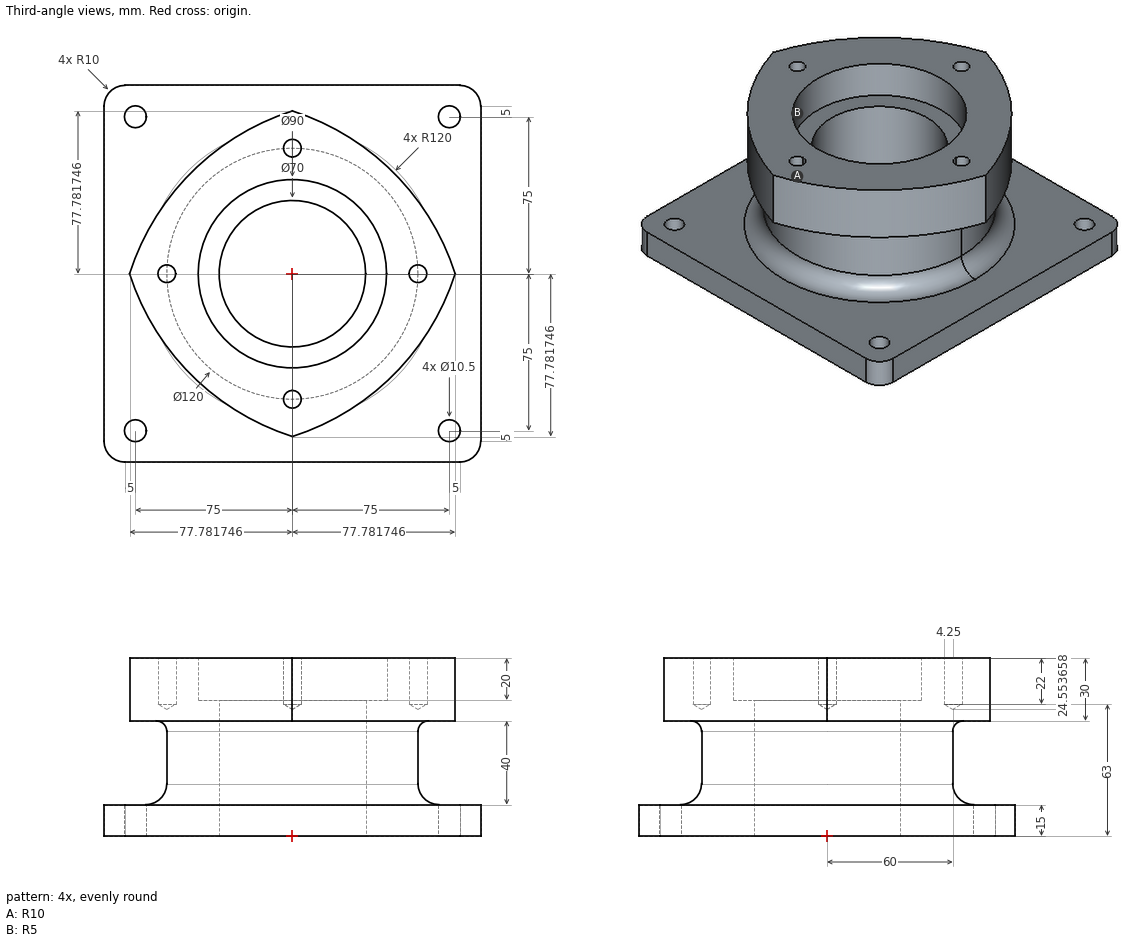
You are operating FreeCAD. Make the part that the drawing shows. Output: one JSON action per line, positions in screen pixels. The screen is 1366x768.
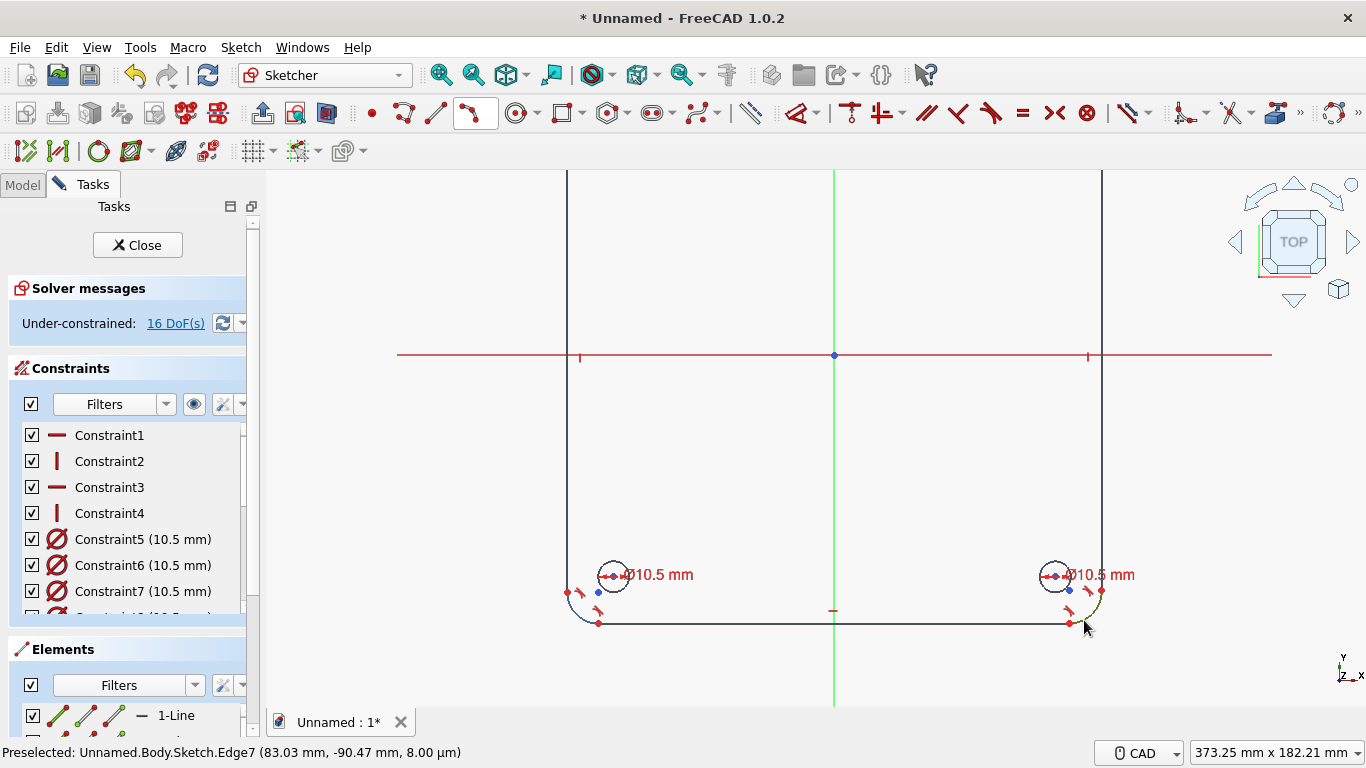
{"action": "scroll", "coordinate": [571, 608], "scroll_direction": "down", "scroll_amount": 2}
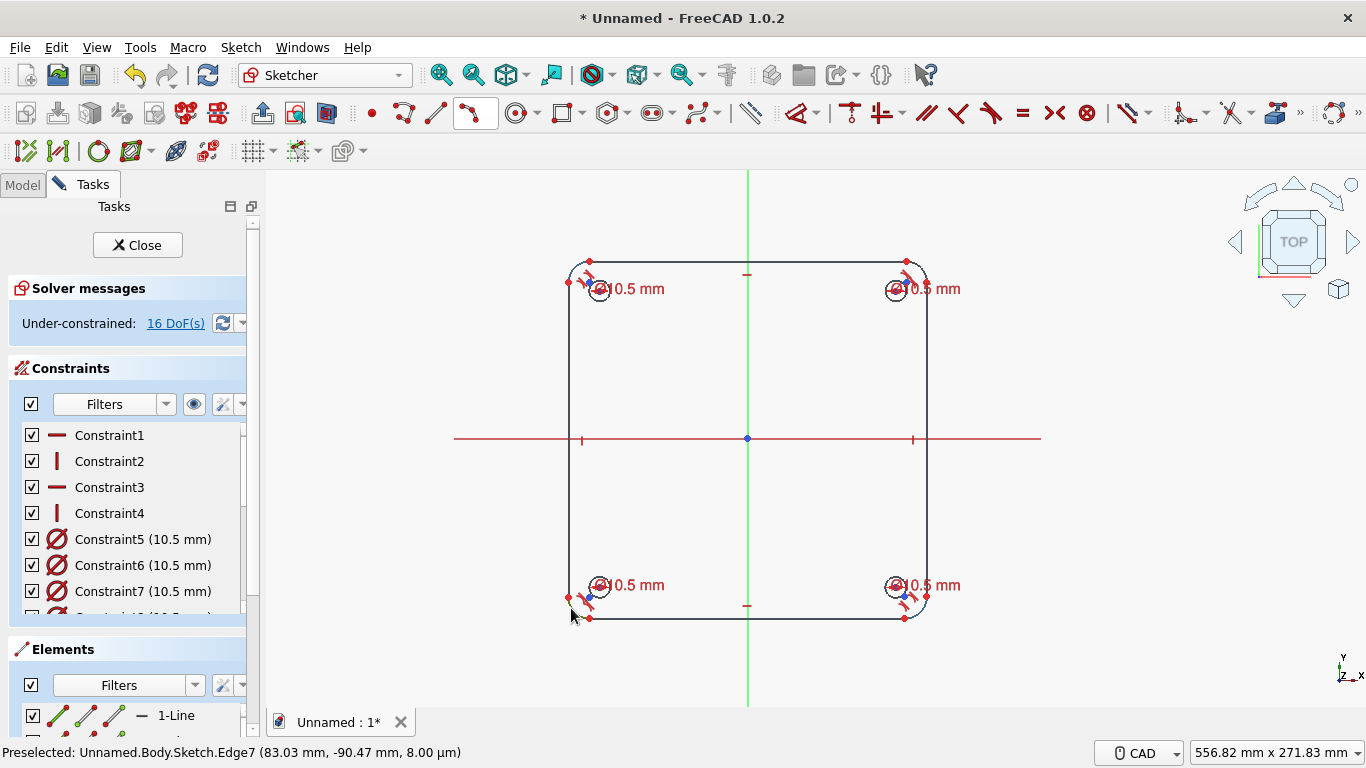
{"action": "scroll", "coordinate": [925, 273], "scroll_direction": "up", "scroll_amount": 2}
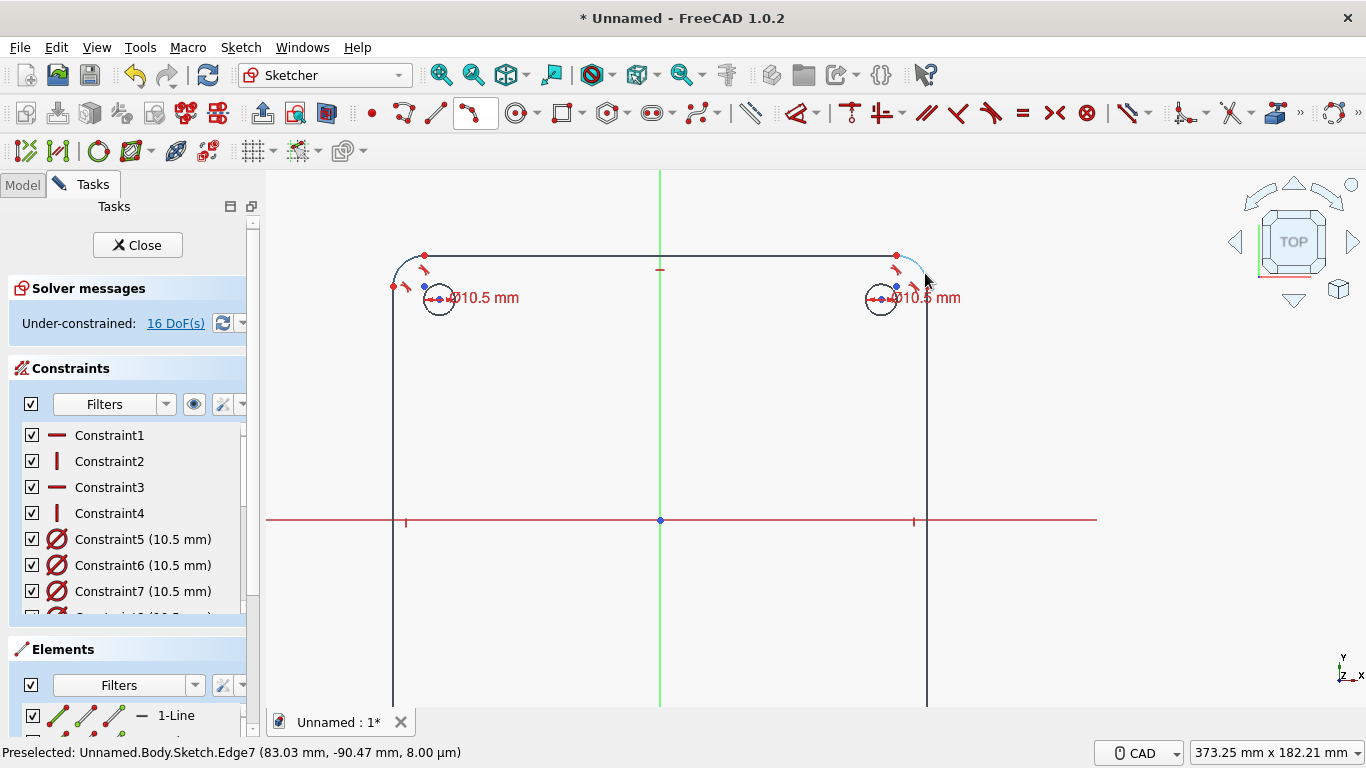
{"action": "left_click", "coordinate": [924, 273]}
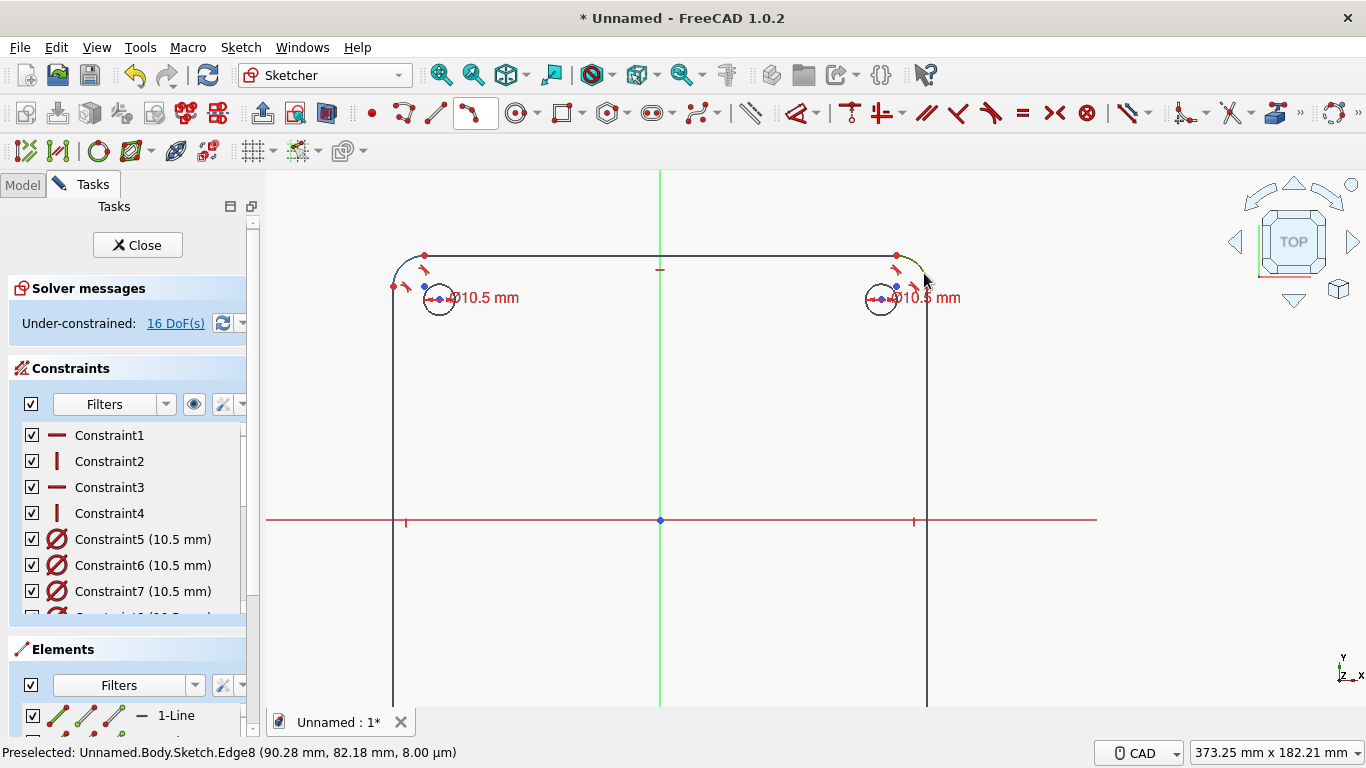
{"action": "left_click", "coordinate": [1024, 114]}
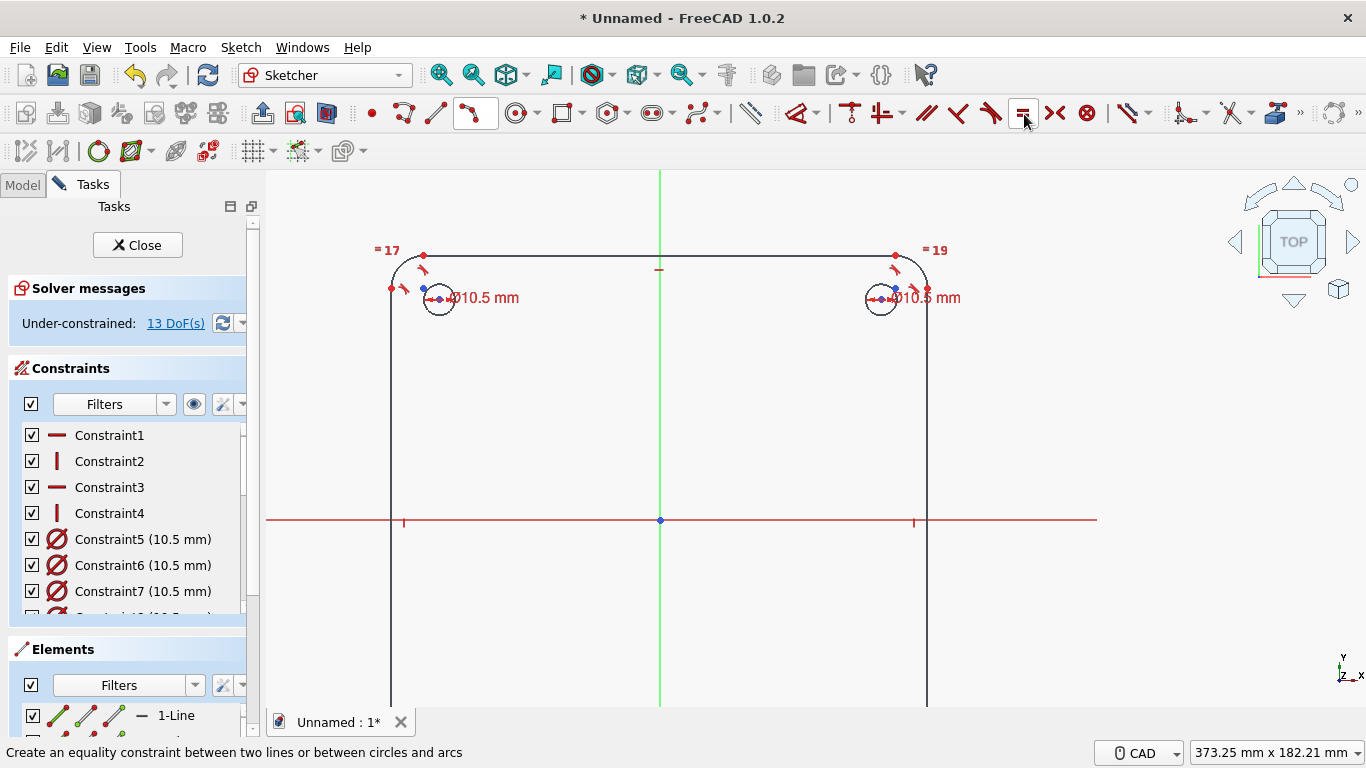
{"action": "scroll", "coordinate": [925, 272], "scroll_direction": "down", "scroll_amount": 2}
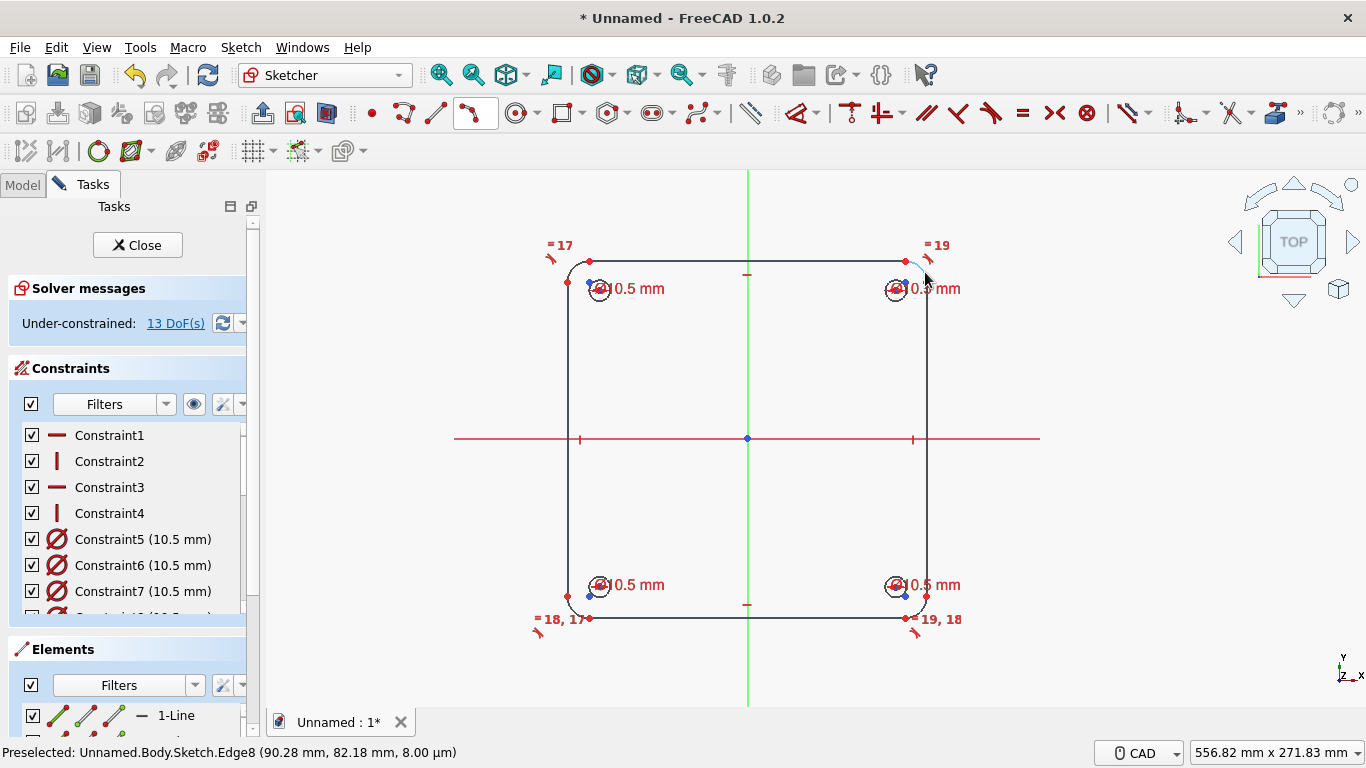
{"action": "left_click", "coordinate": [896, 587]}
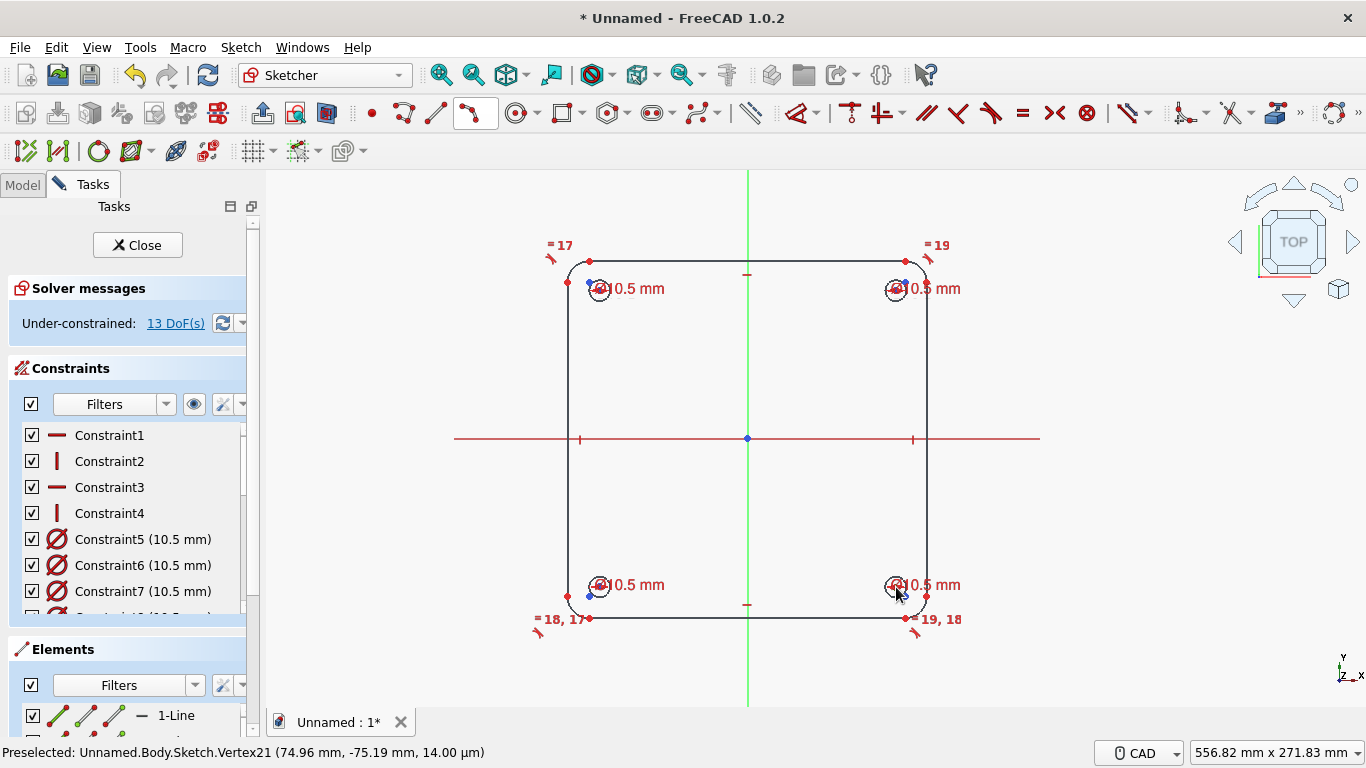
{"action": "left_click", "coordinate": [600, 587]}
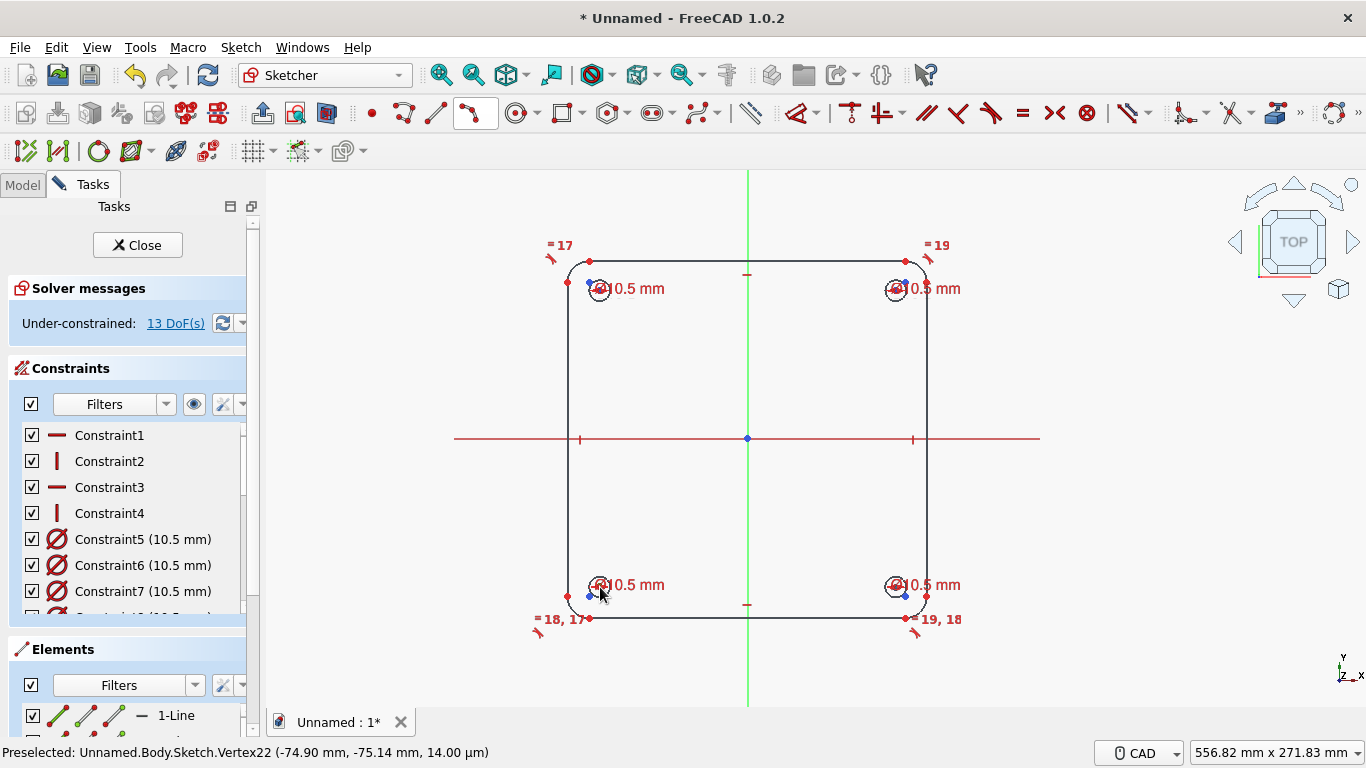
{"action": "left_click", "coordinate": [904, 114]}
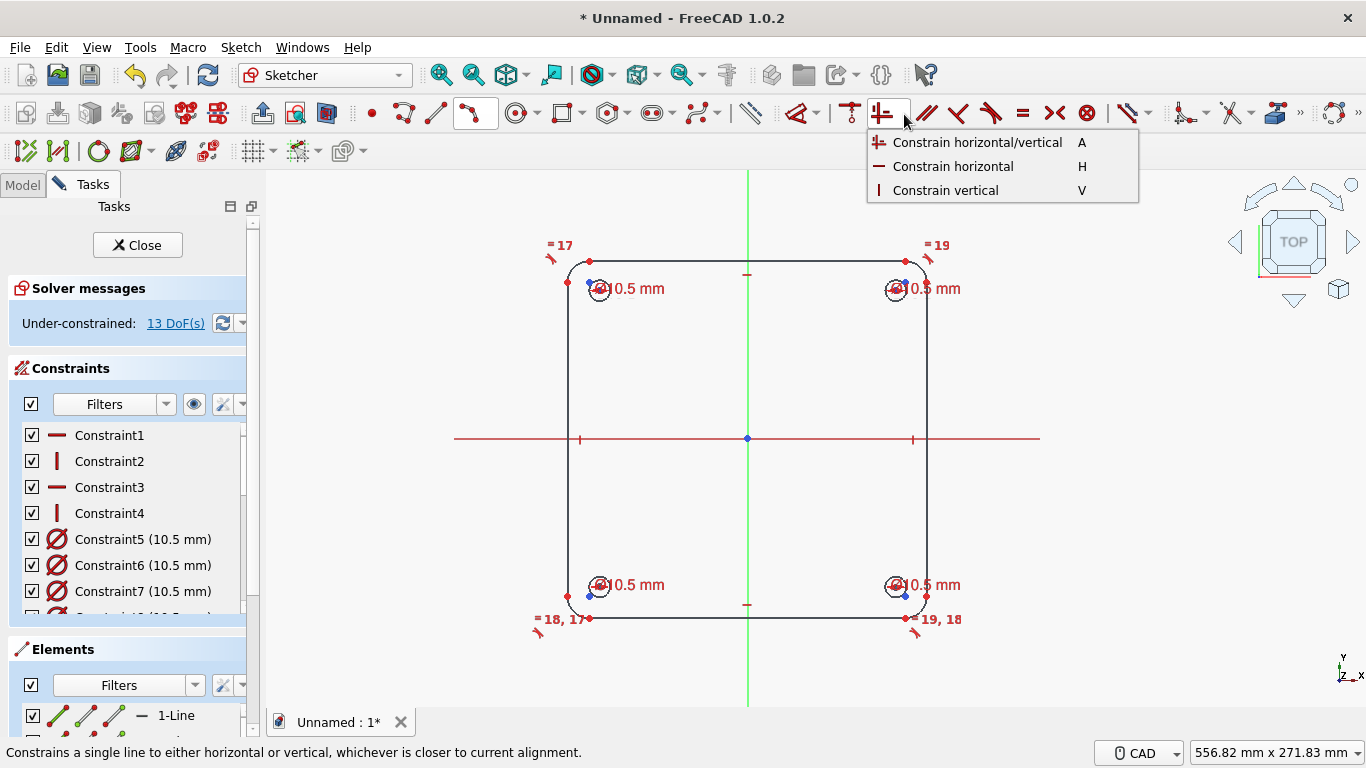
{"action": "left_click", "coordinate": [1003, 166]}